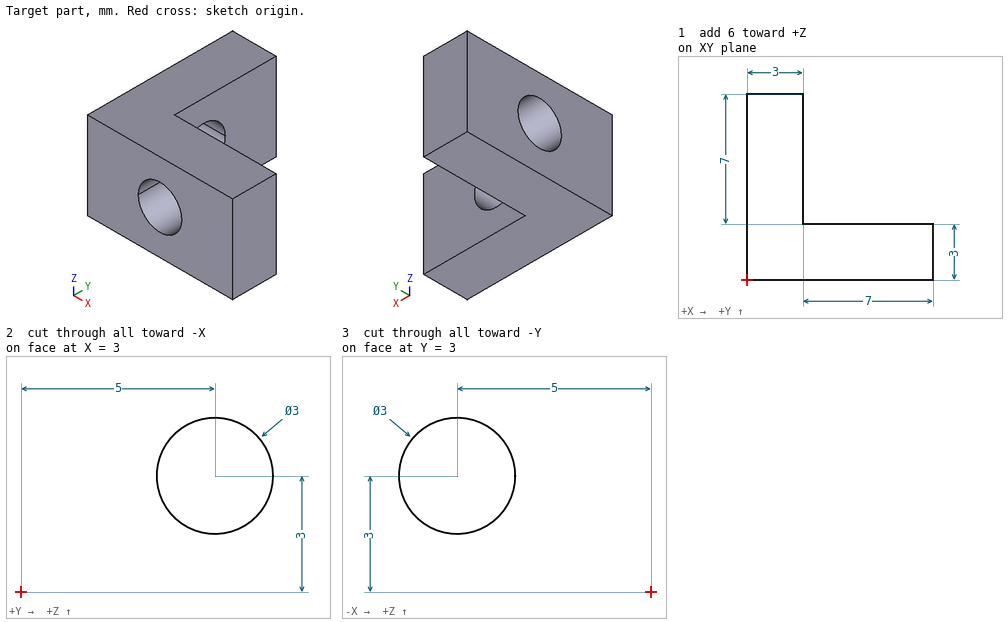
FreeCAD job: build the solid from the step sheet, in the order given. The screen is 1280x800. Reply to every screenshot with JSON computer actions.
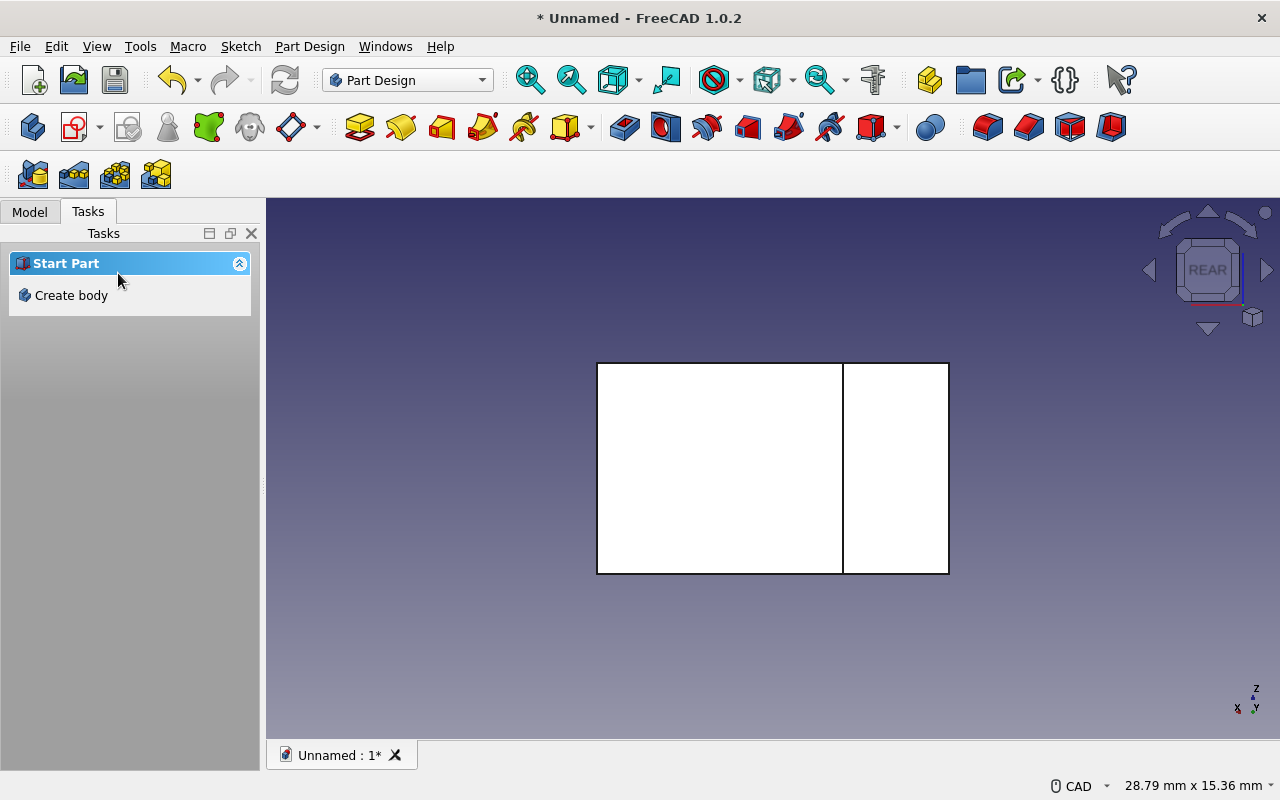
{"action": "left_click", "coordinate": [531, 80]}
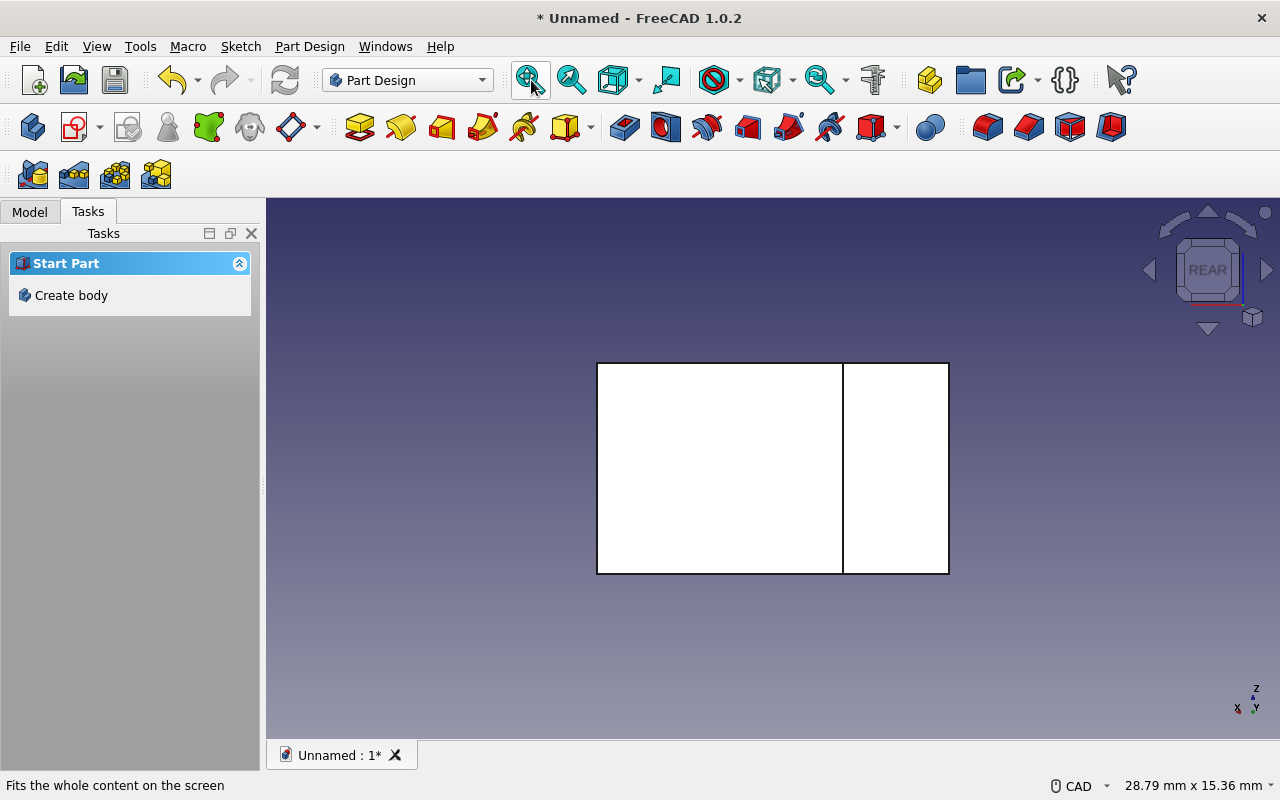
{"action": "left_click", "coordinate": [720, 468]}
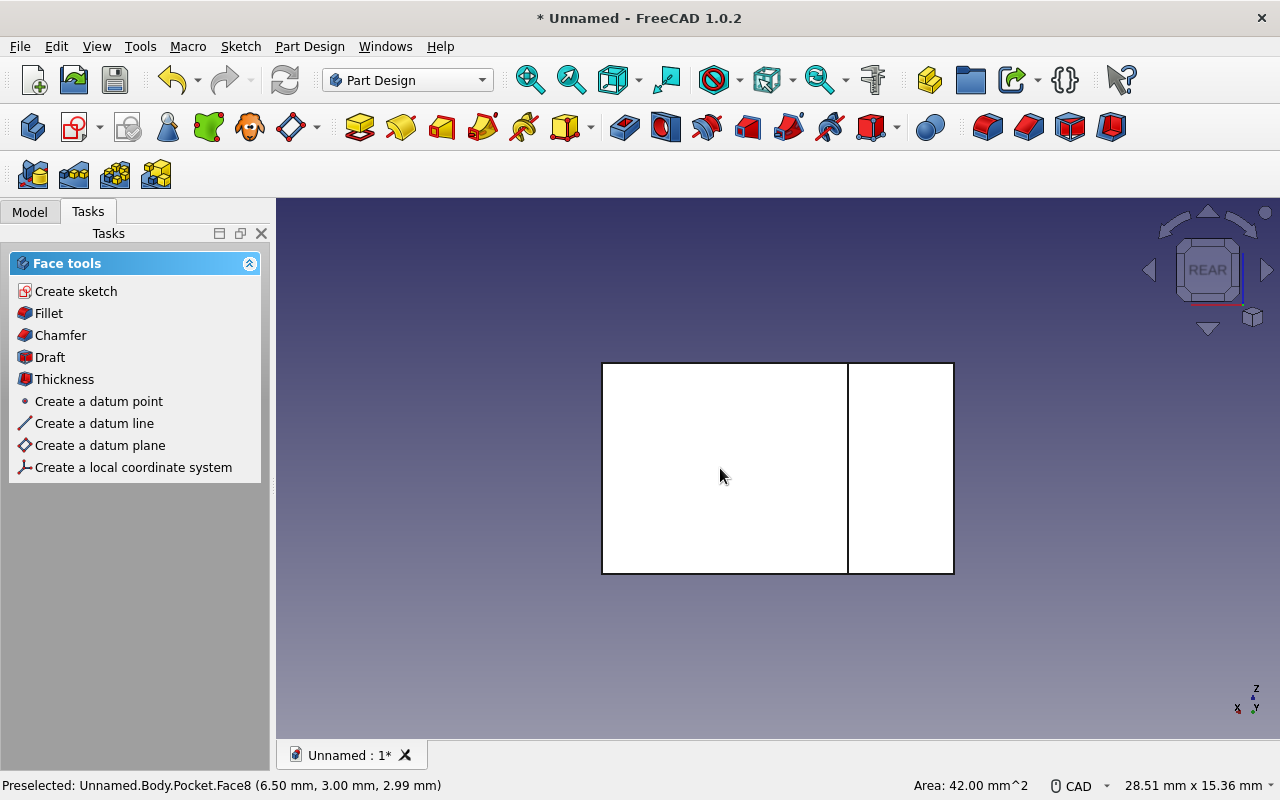
{"action": "left_click", "coordinate": [74, 128]}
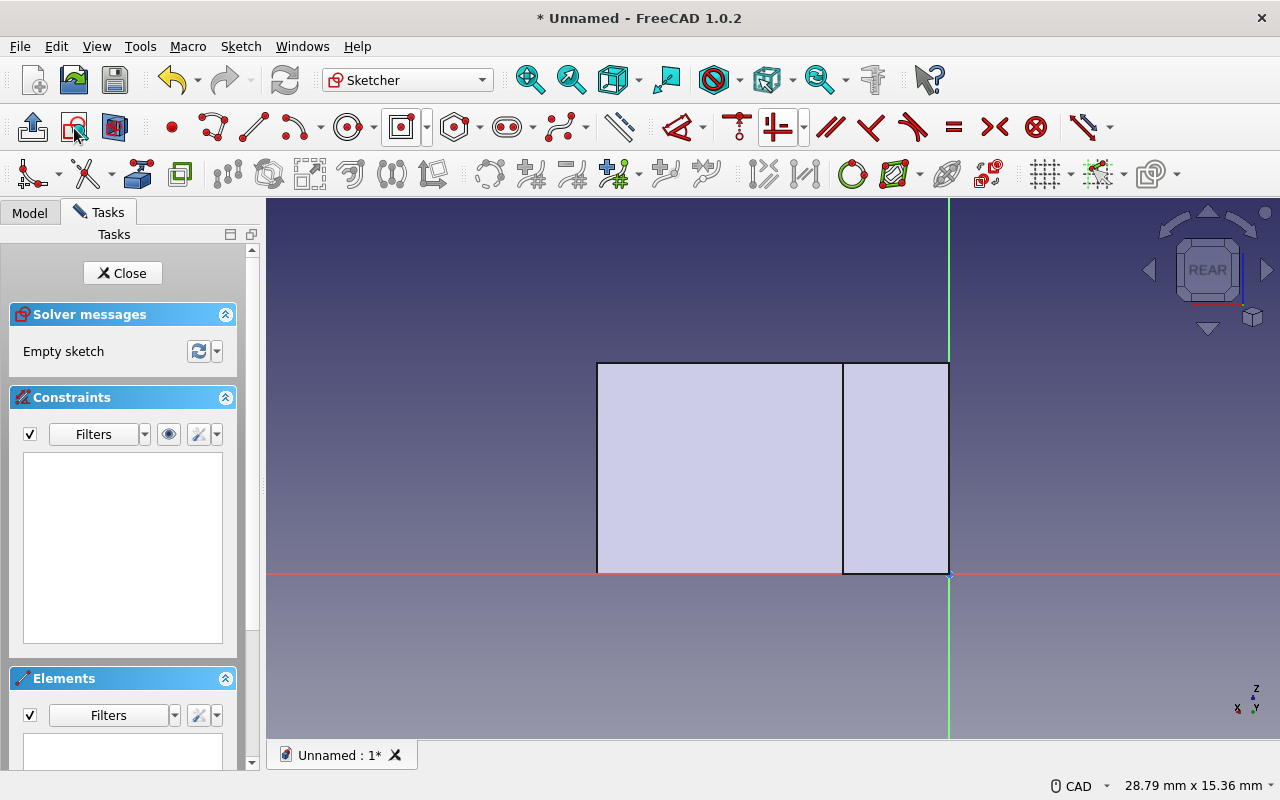
{"action": "scroll", "coordinate": [941, 516], "scroll_direction": "up", "scroll_amount": 4}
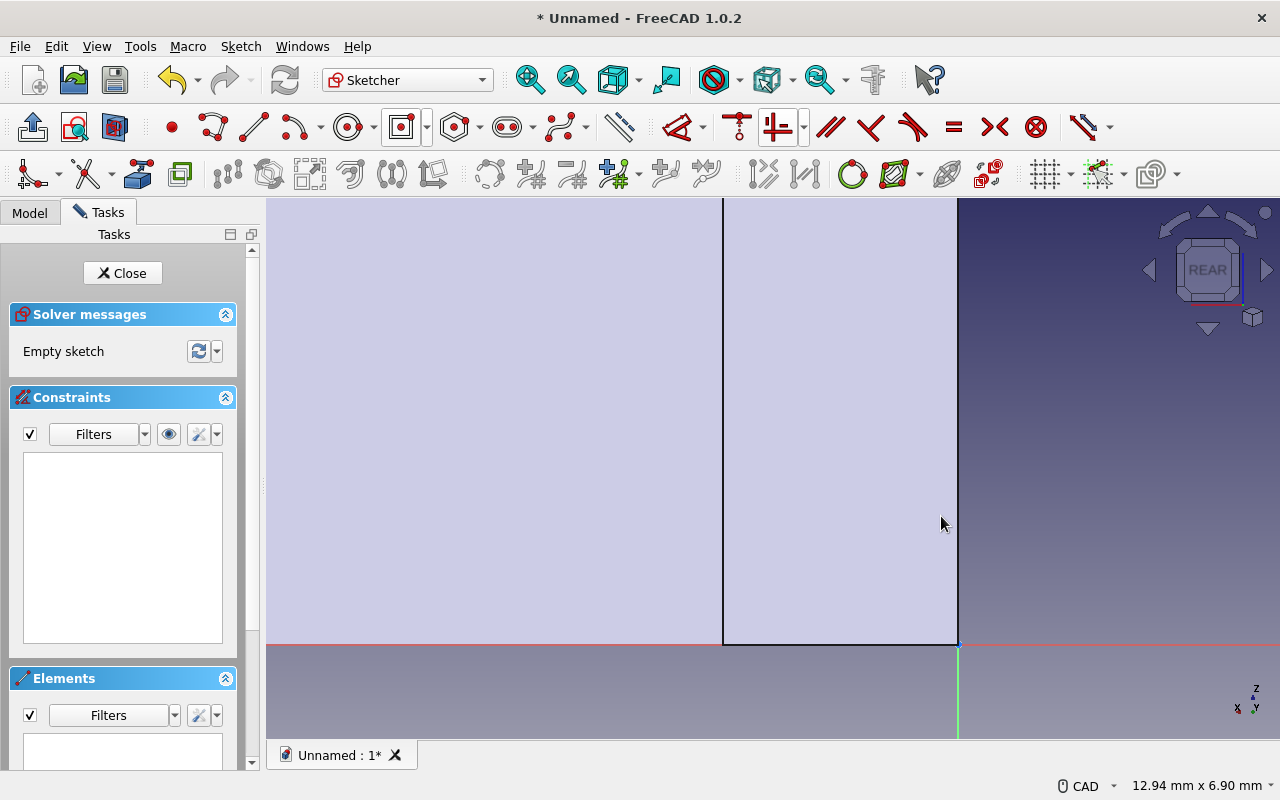
{"action": "left_click", "coordinate": [348, 128]}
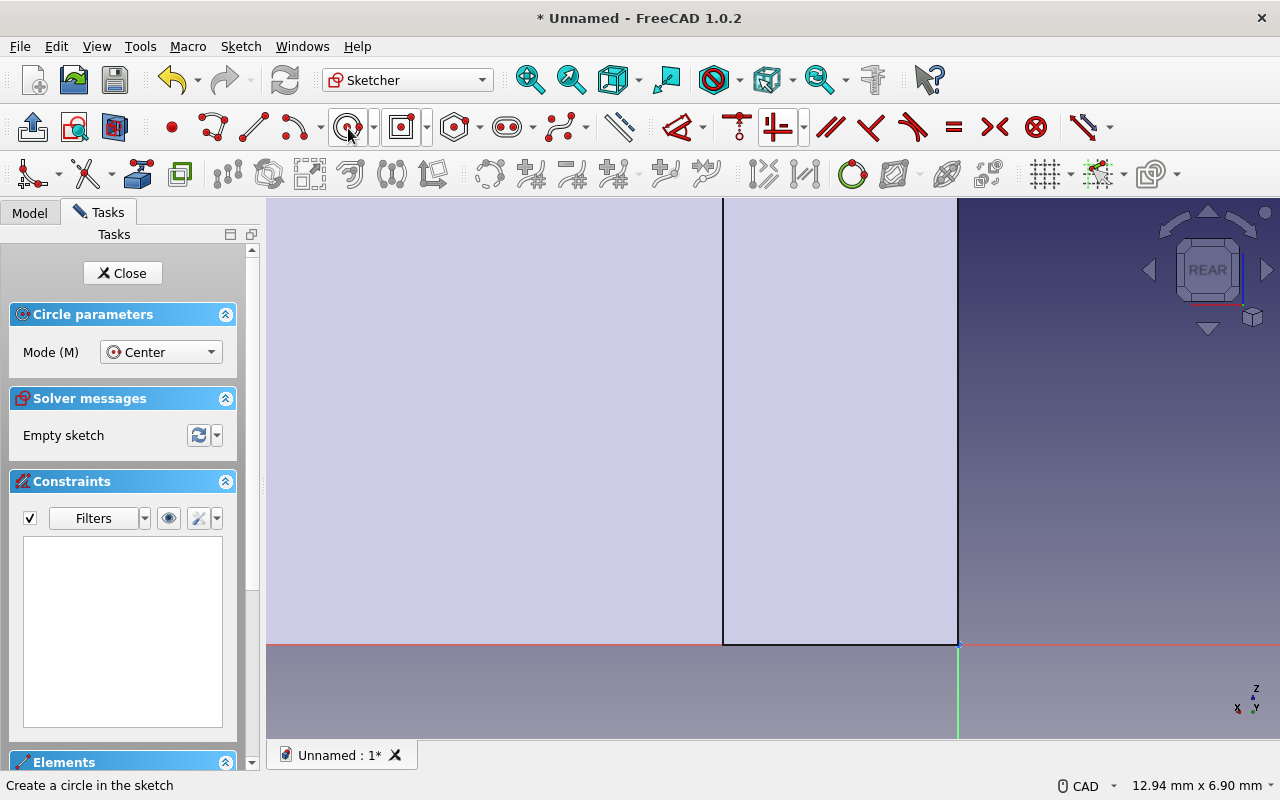
{"action": "left_click", "coordinate": [566, 410]}
{"action": "left_click", "coordinate": [649, 326]}
{"action": "key", "text": "Escape"}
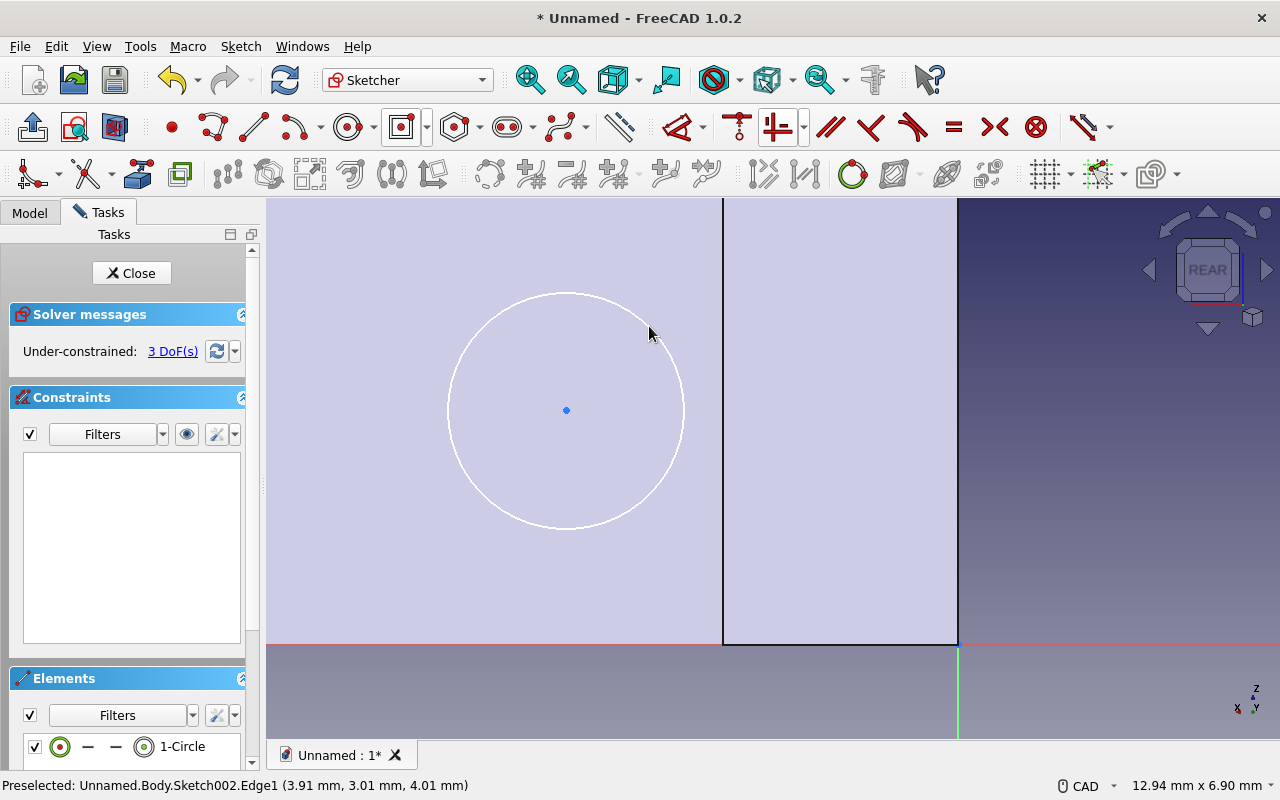
{"action": "left_click", "coordinate": [676, 128]}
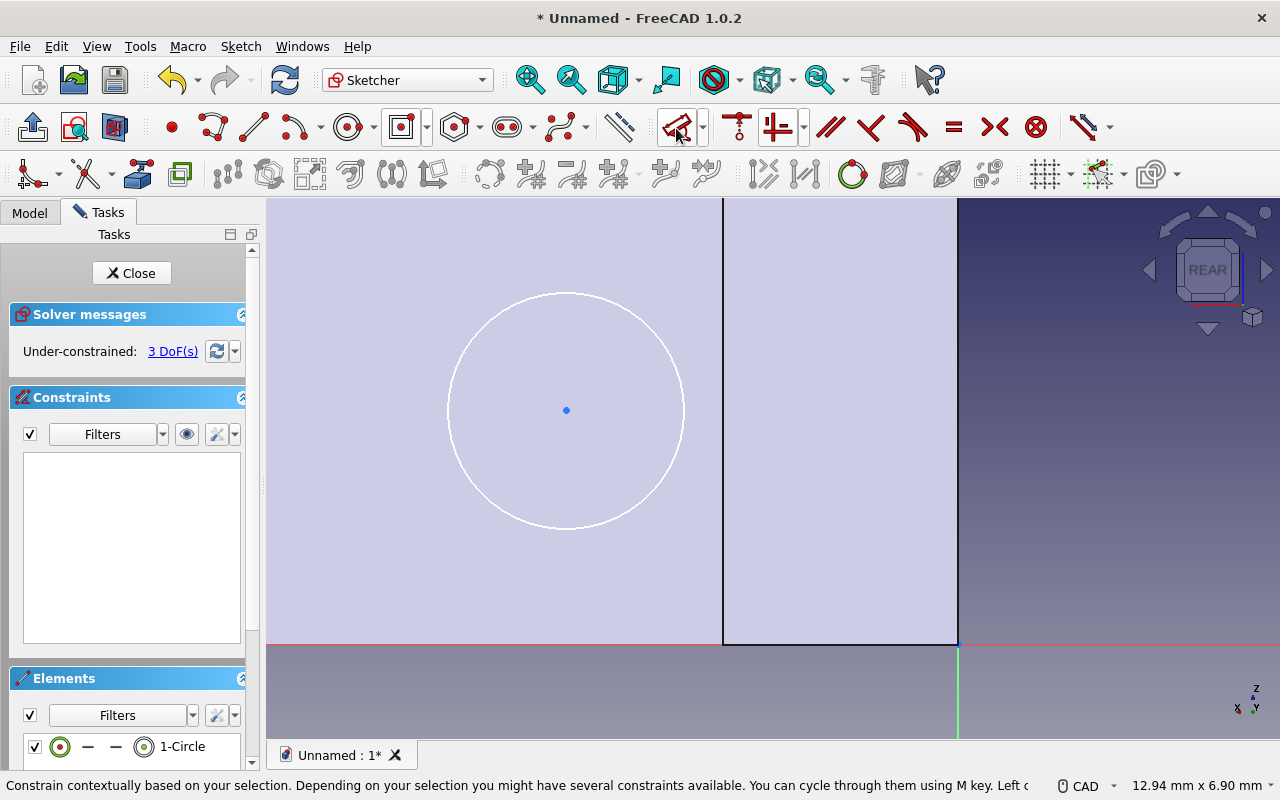
{"action": "left_click", "coordinate": [649, 327]}
{"action": "left_click", "coordinate": [671, 304]}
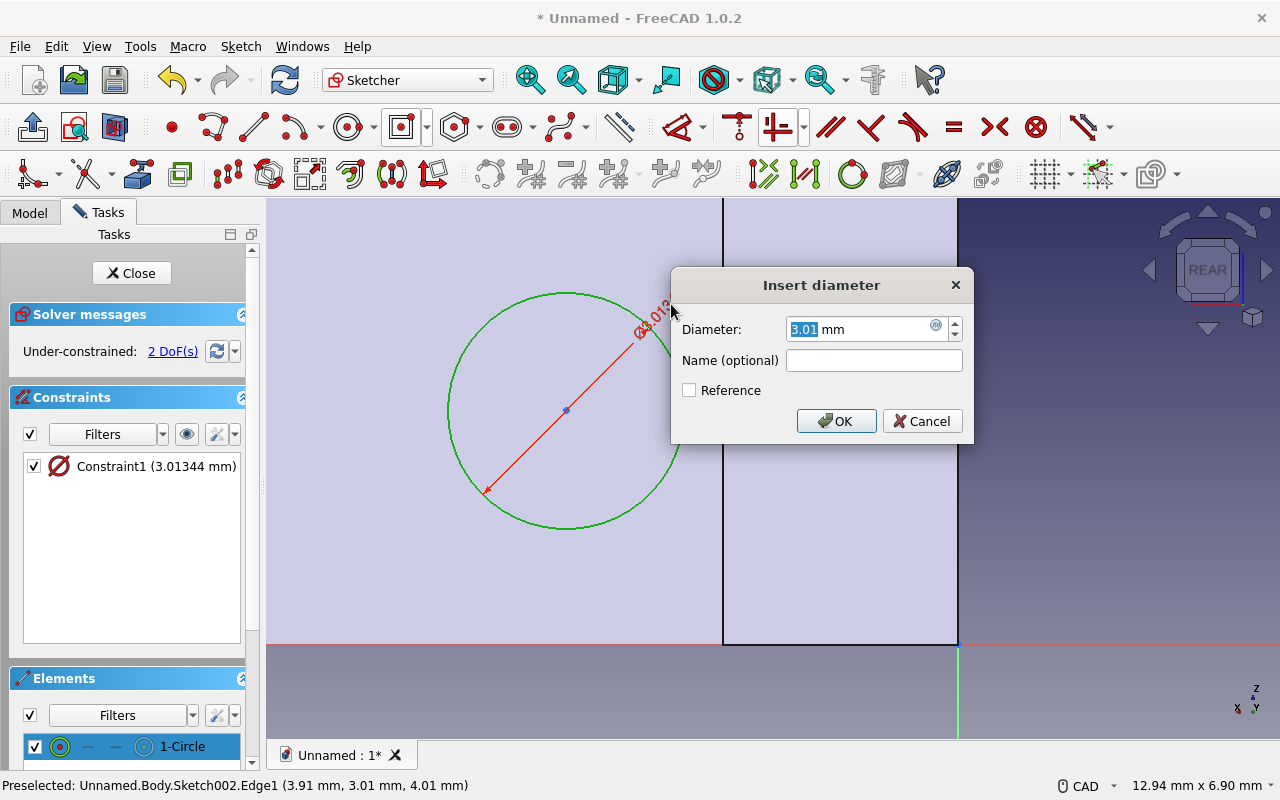
{"action": "type", "text": "3"}
{"action": "key", "text": "Return"}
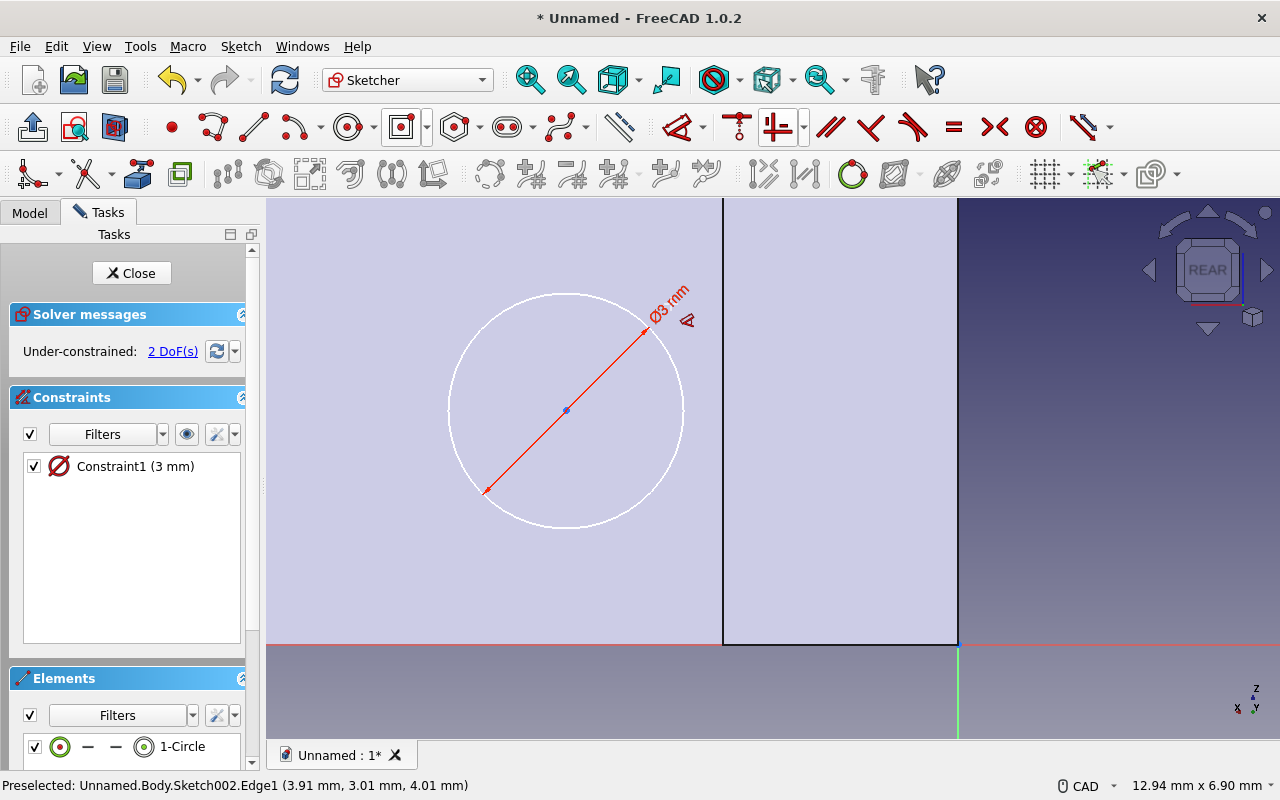
{"action": "left_click", "coordinate": [566, 411]}
{"action": "left_click", "coordinate": [762, 679]}